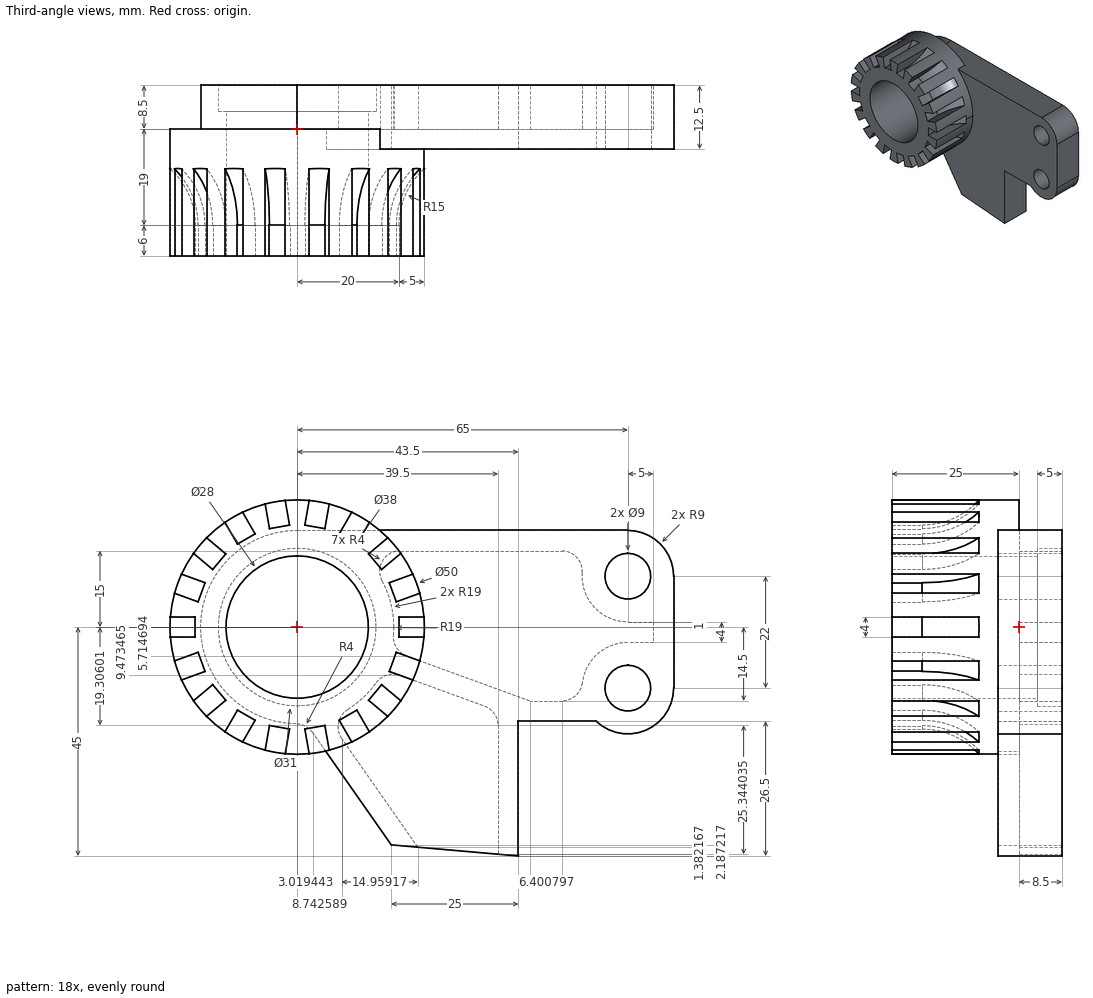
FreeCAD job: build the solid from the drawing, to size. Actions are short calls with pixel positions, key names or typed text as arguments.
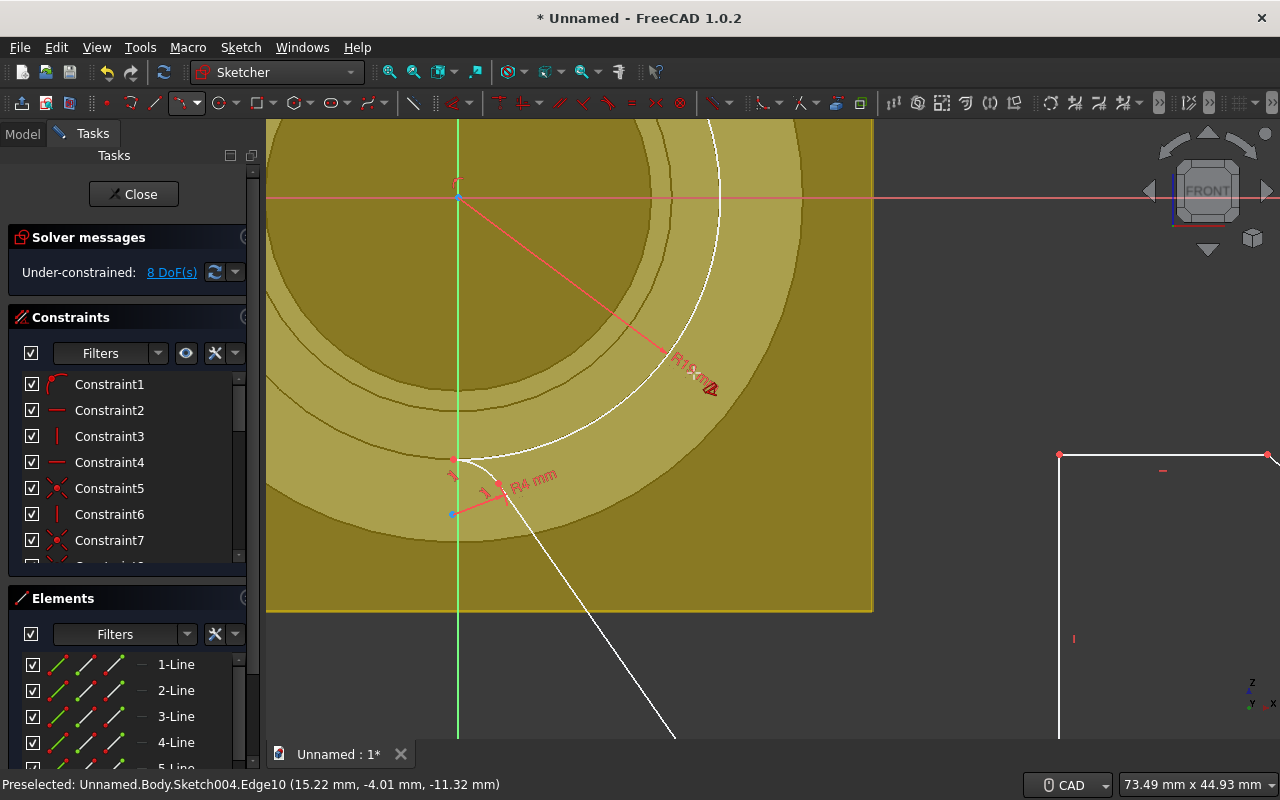
scroll(490, 471, down, 4)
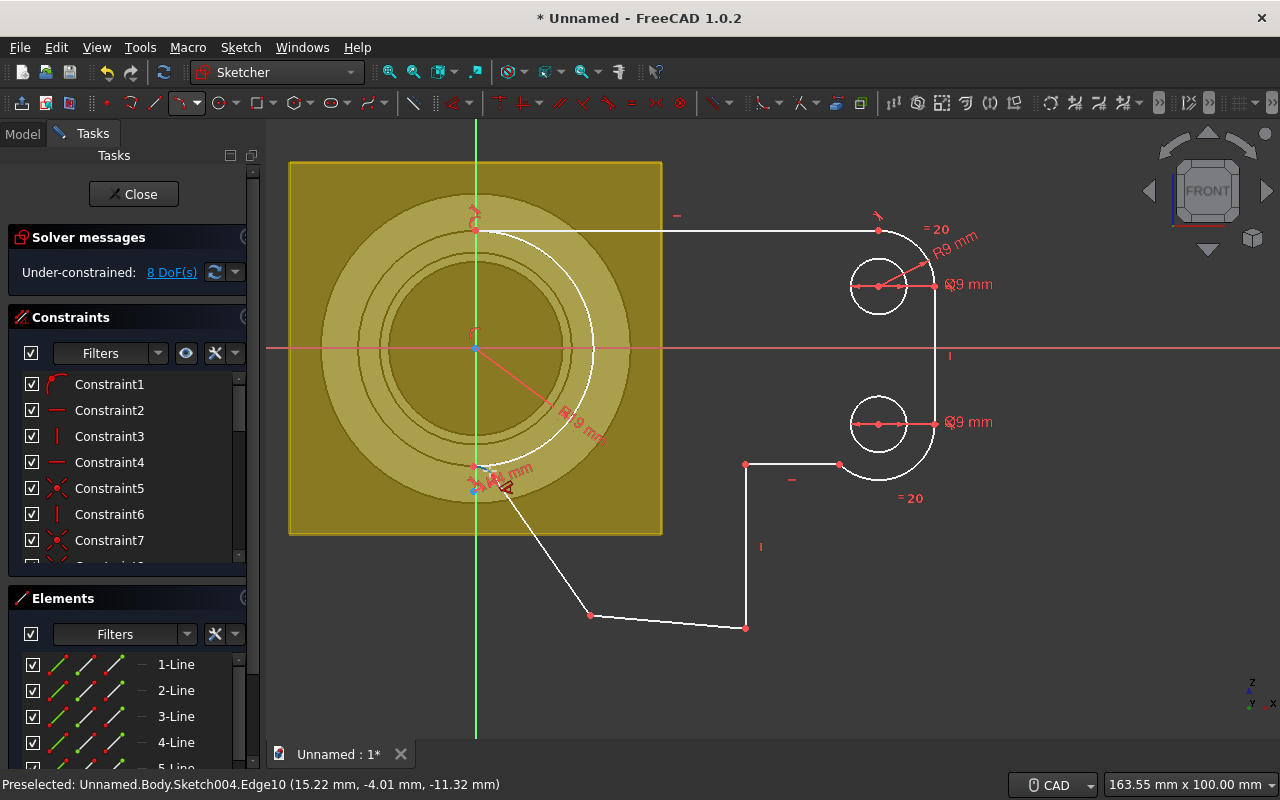
click(597, 231)
click(677, 197)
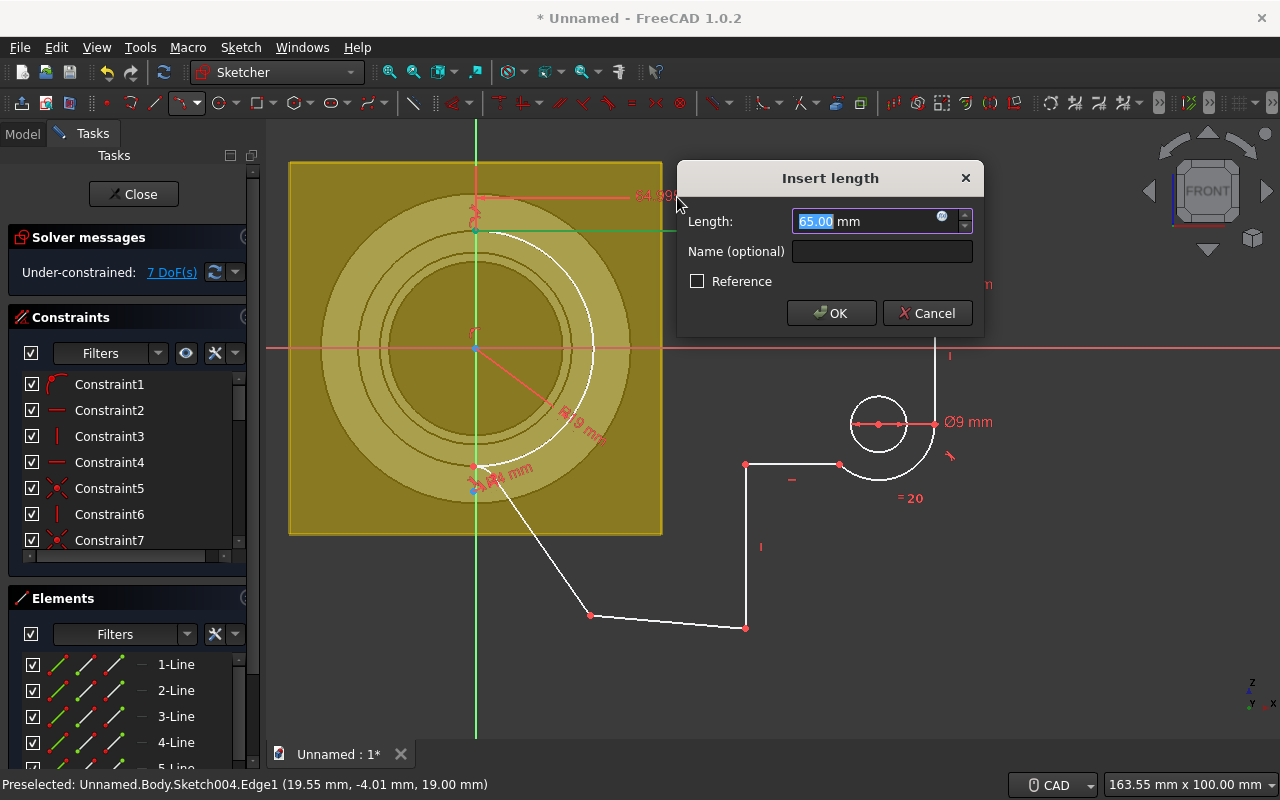
text(65)
key(Return)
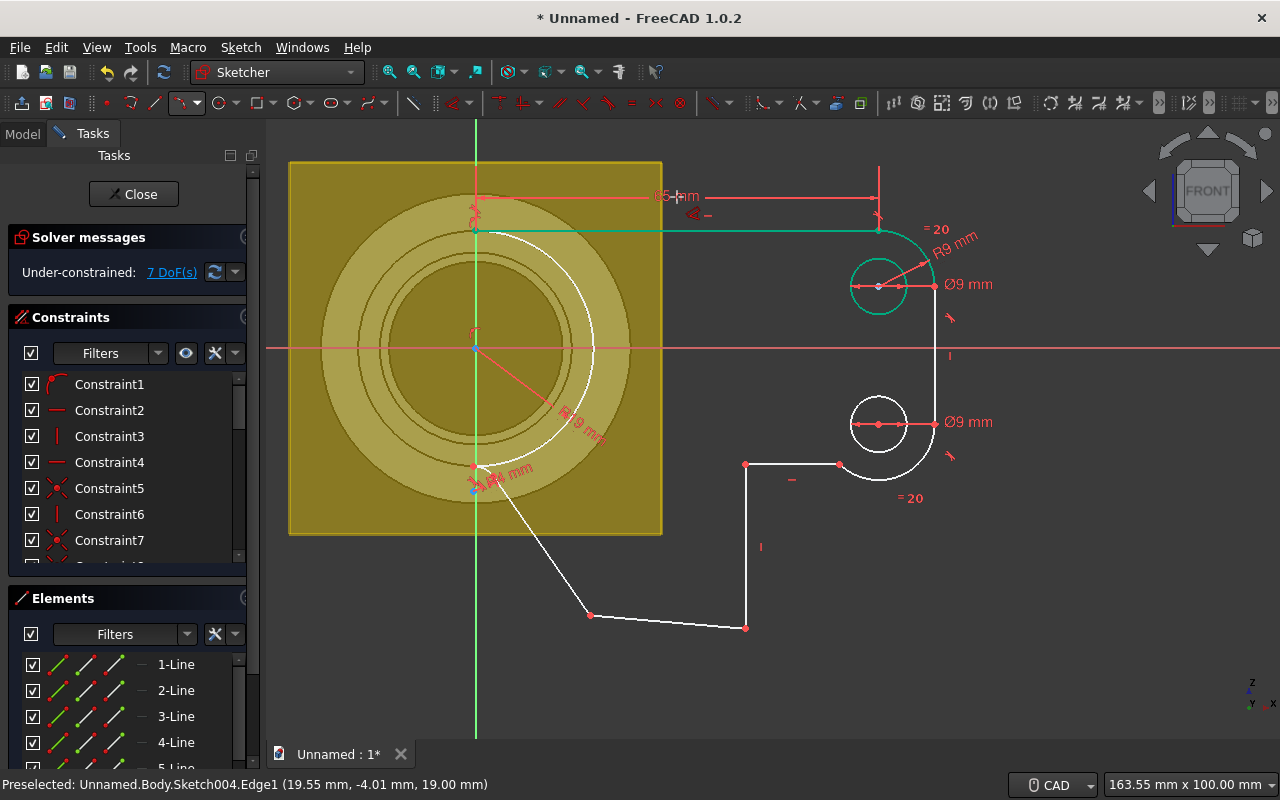
click(935, 328)
click(969, 324)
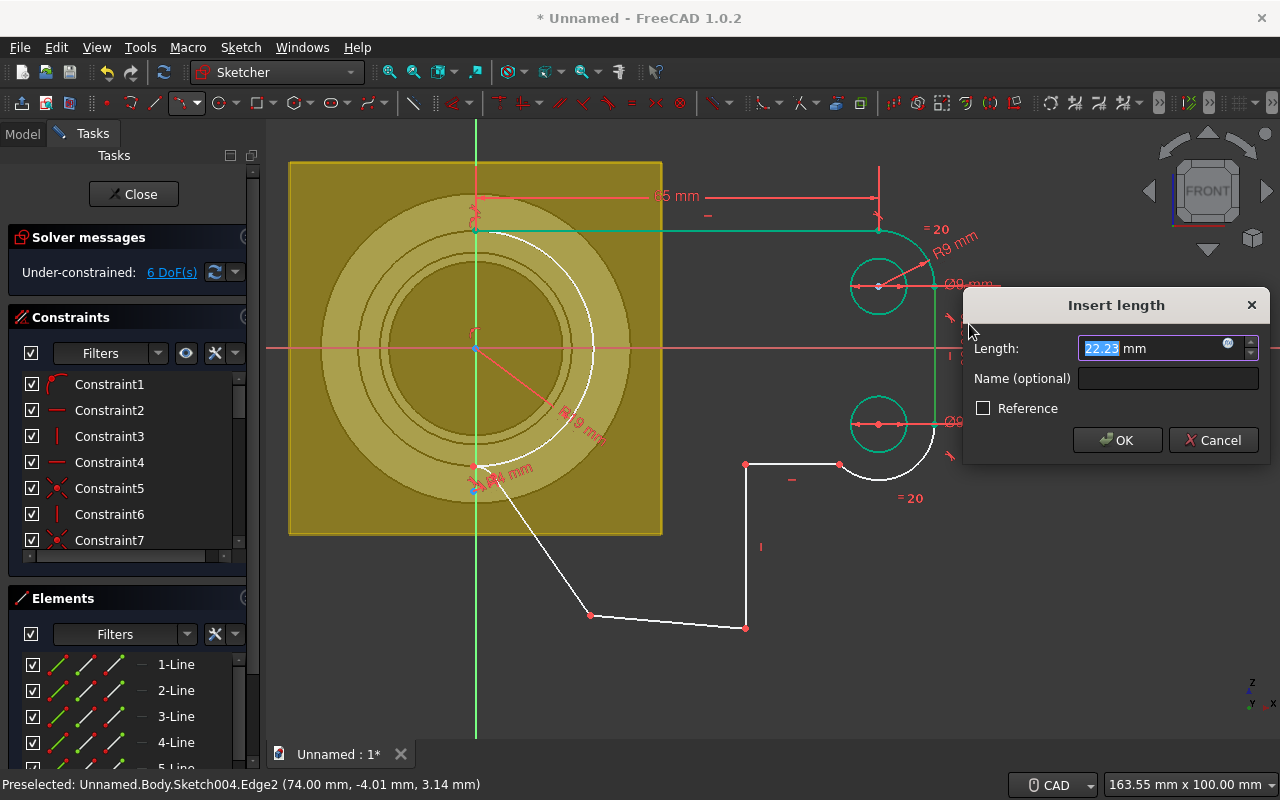
text(22)
key(Return)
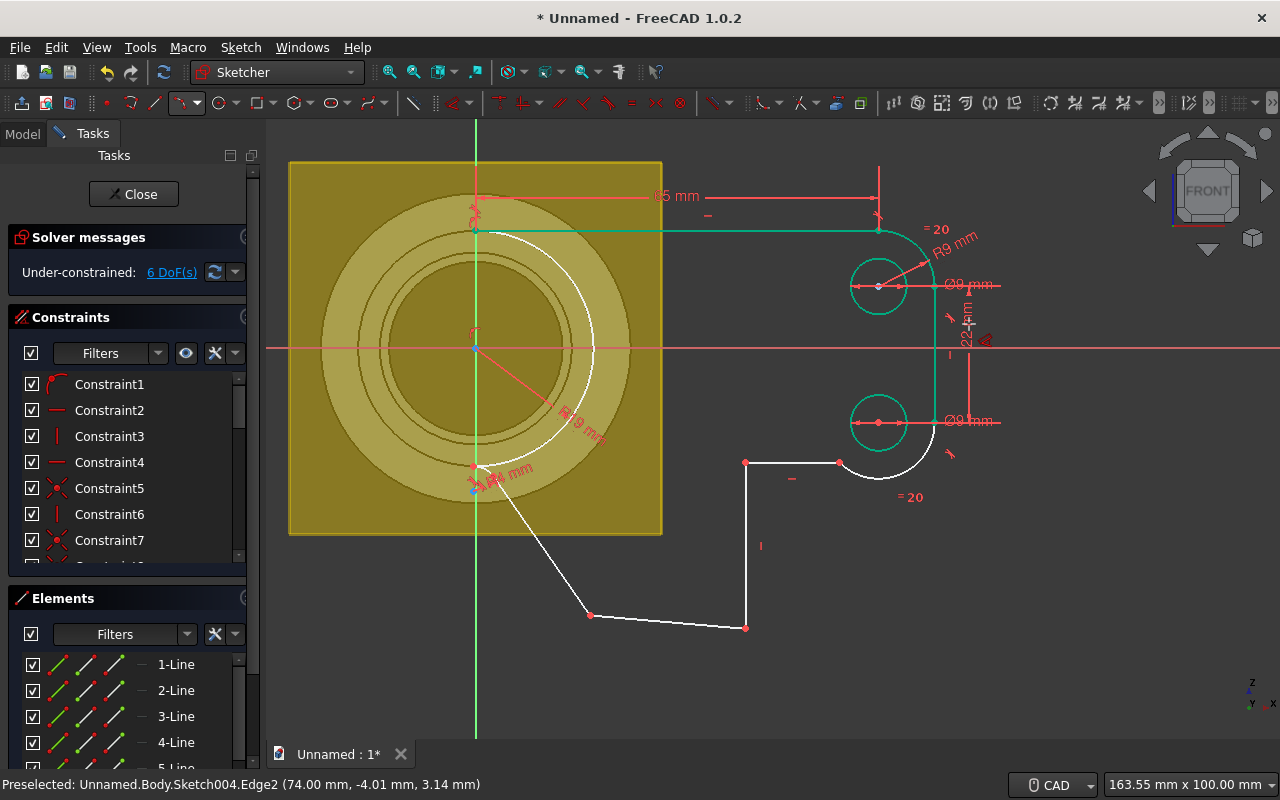
click(746, 629)
click(442, 424)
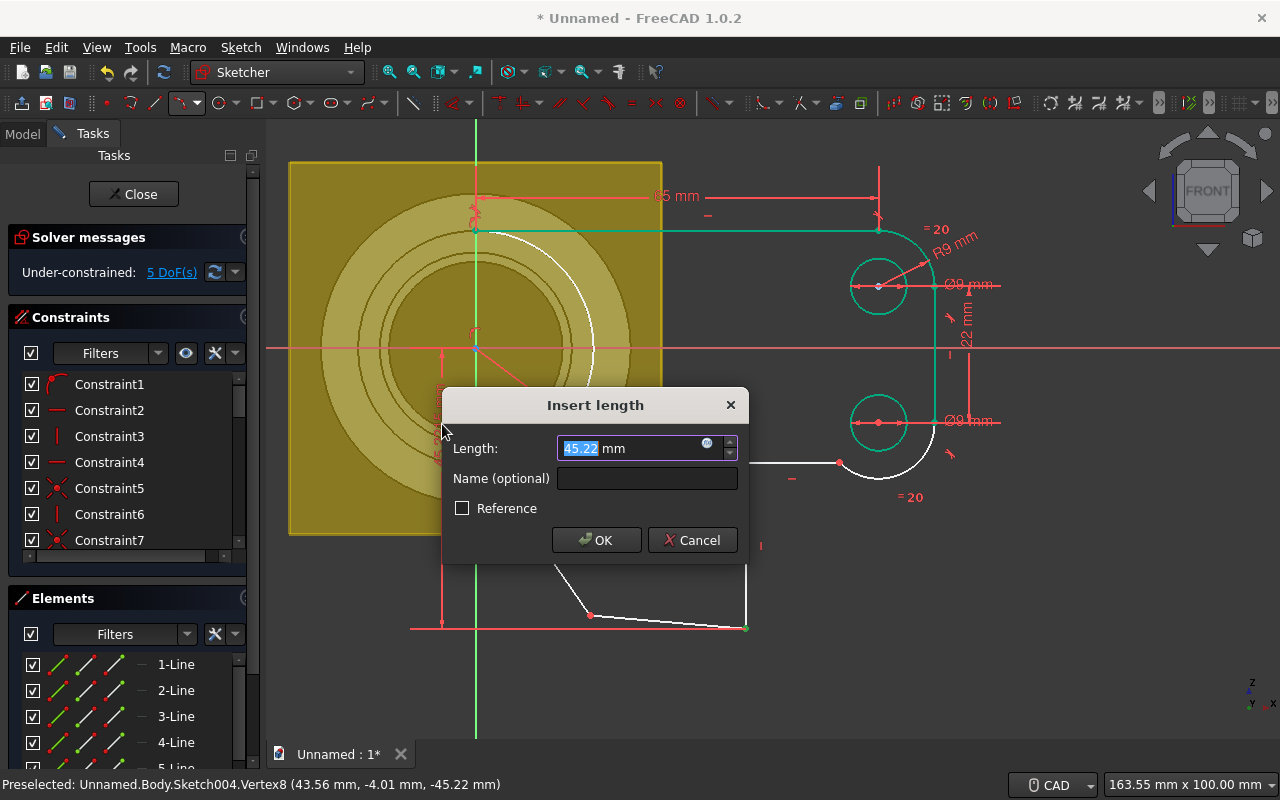
text(45)
key(Return)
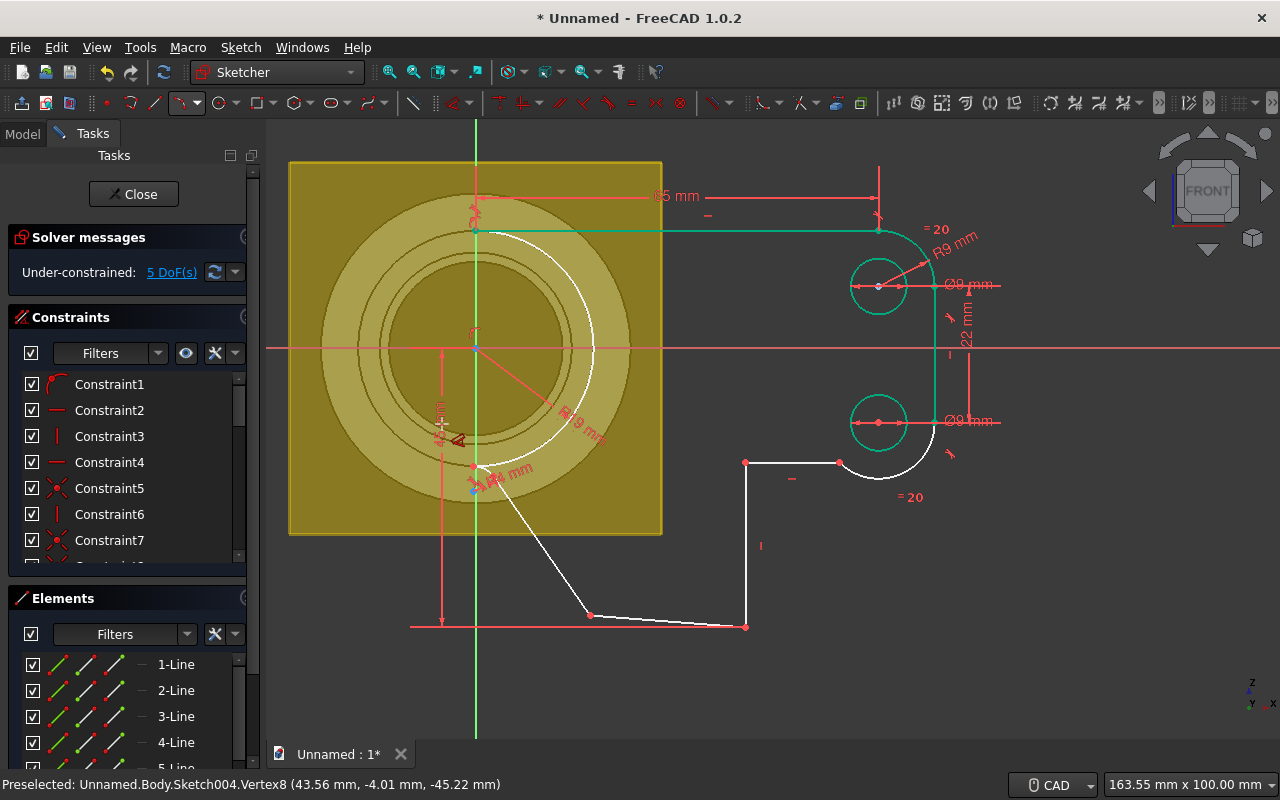
click(699, 624)
click(668, 661)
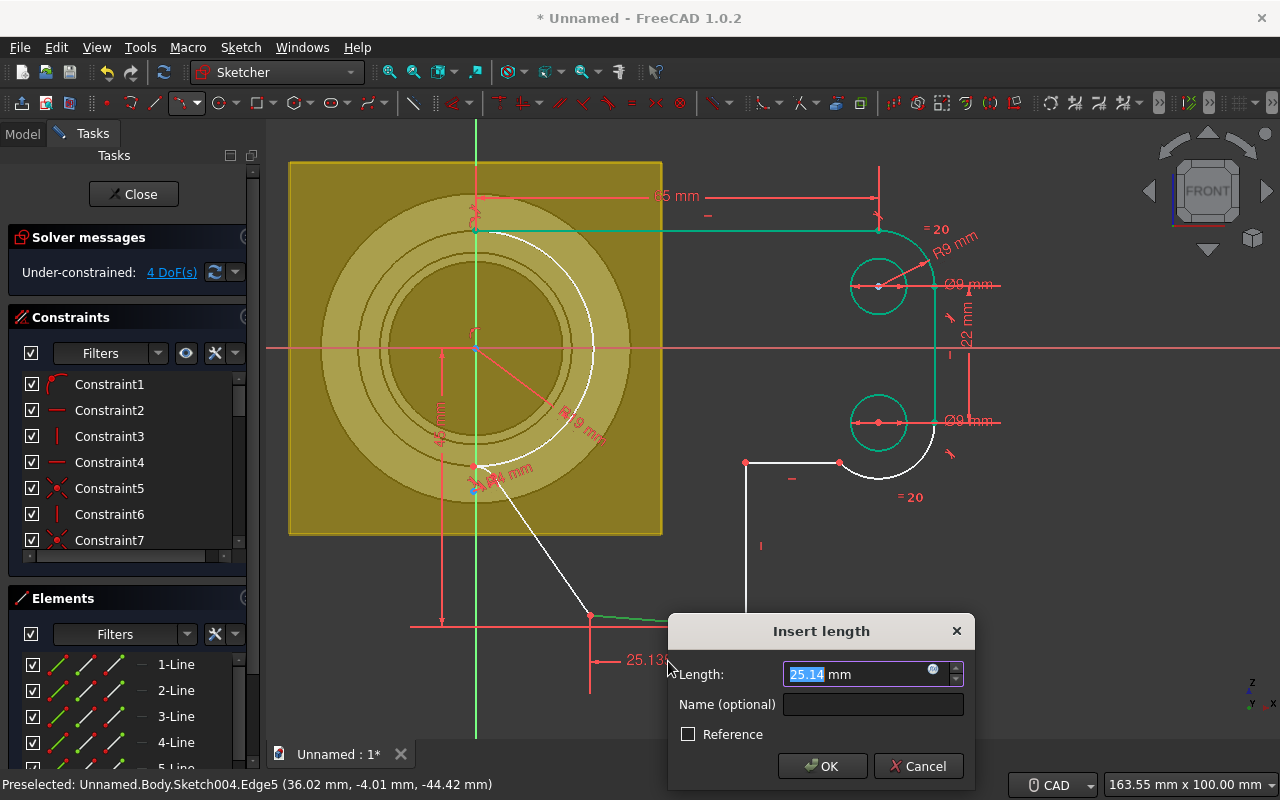
text(25)
key(Return)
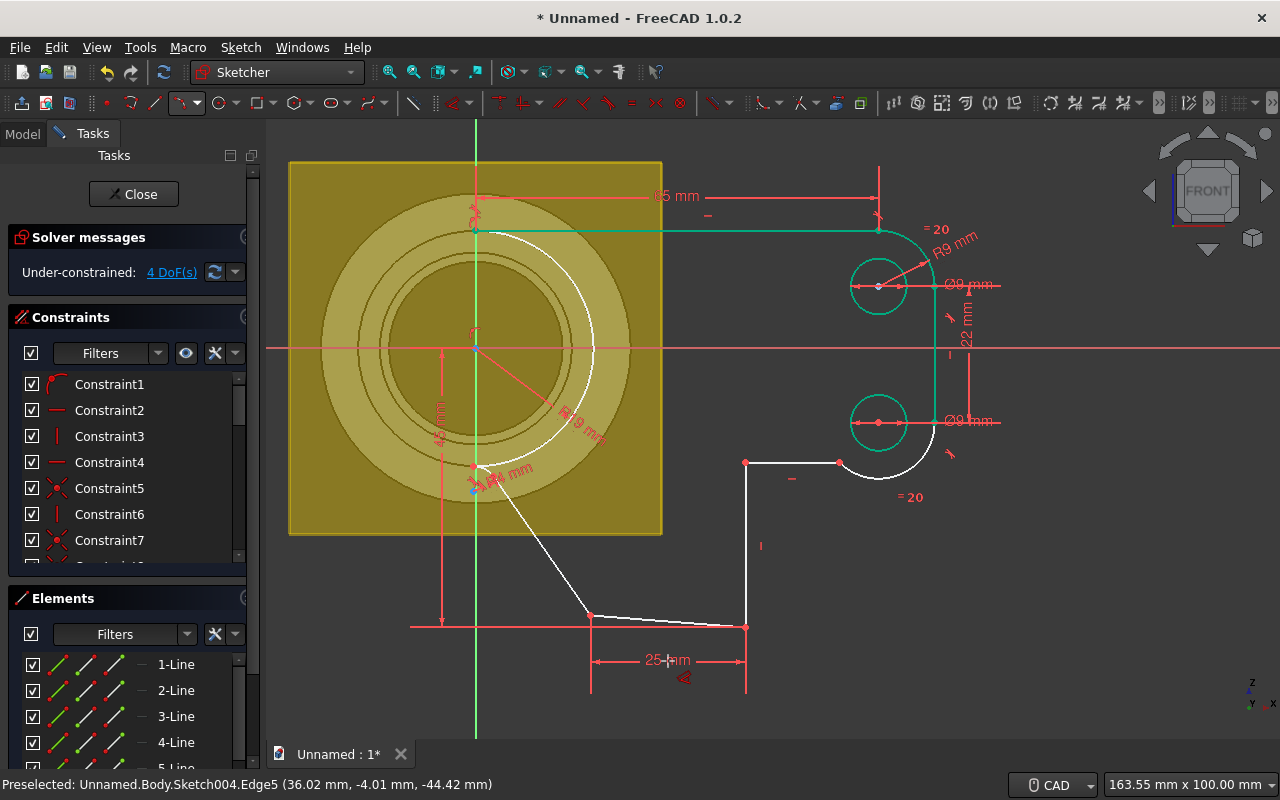
click(746, 512)
click(780, 545)